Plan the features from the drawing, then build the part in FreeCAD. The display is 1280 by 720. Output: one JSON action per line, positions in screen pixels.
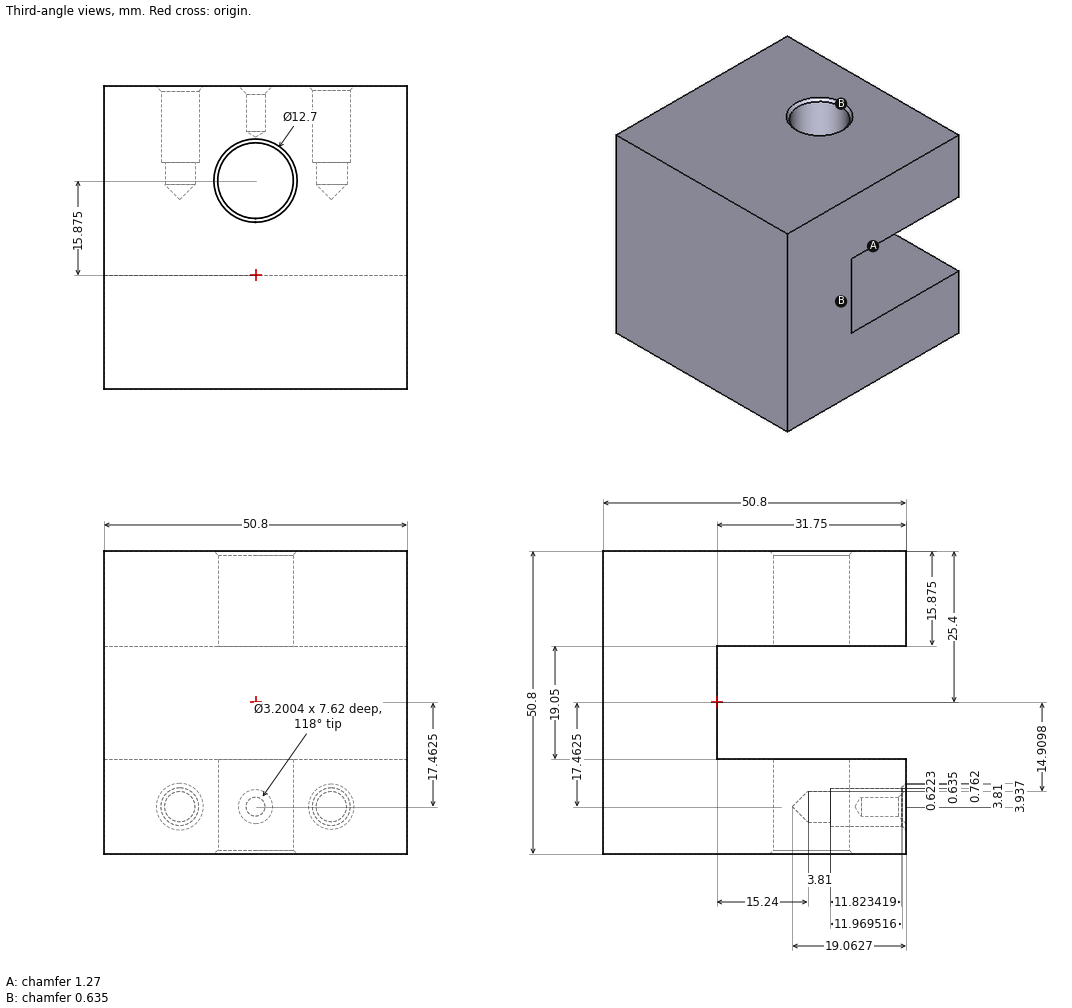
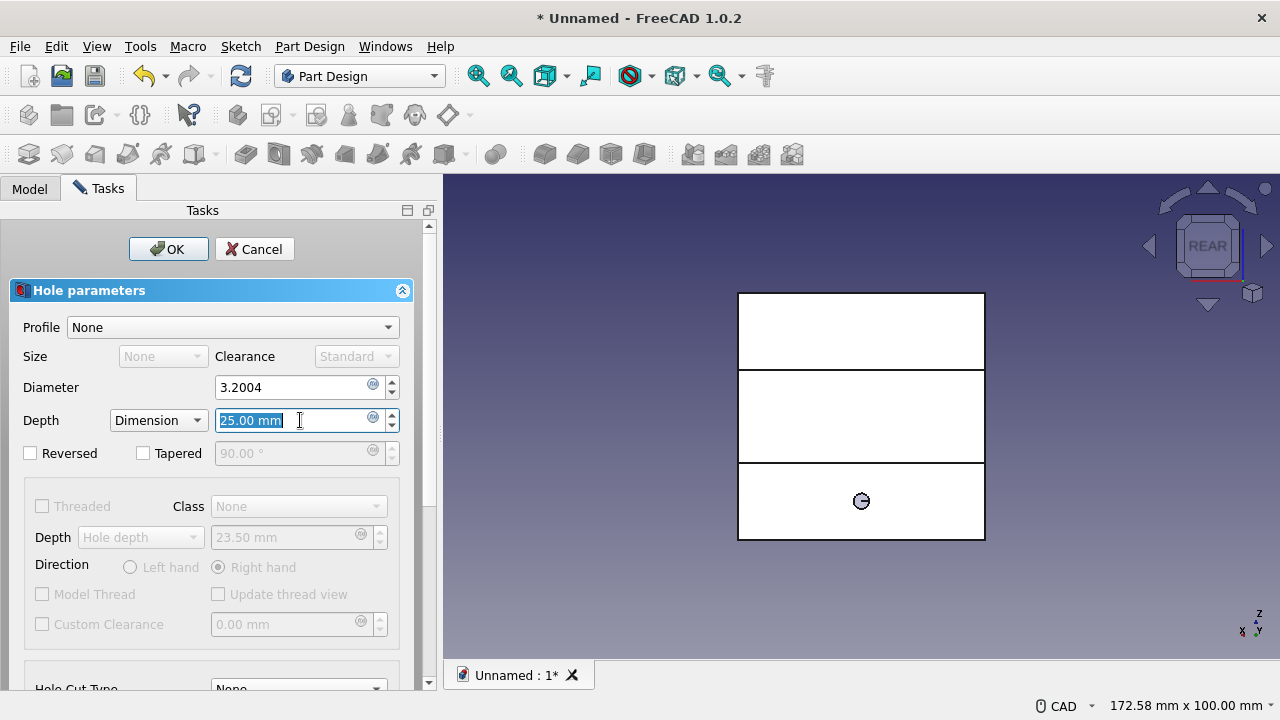
{"action": "type", "text": "7.62"}
{"action": "key", "text": "Tab"}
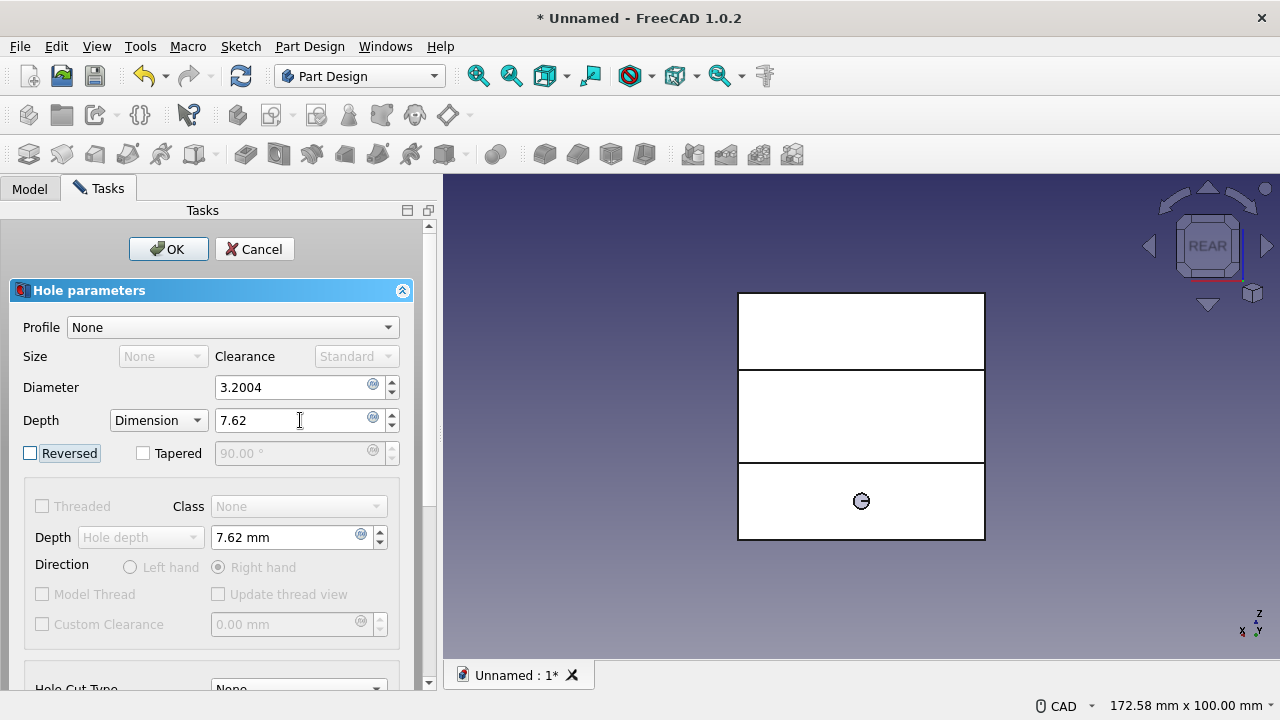
{"action": "left_click", "coordinate": [169, 249]}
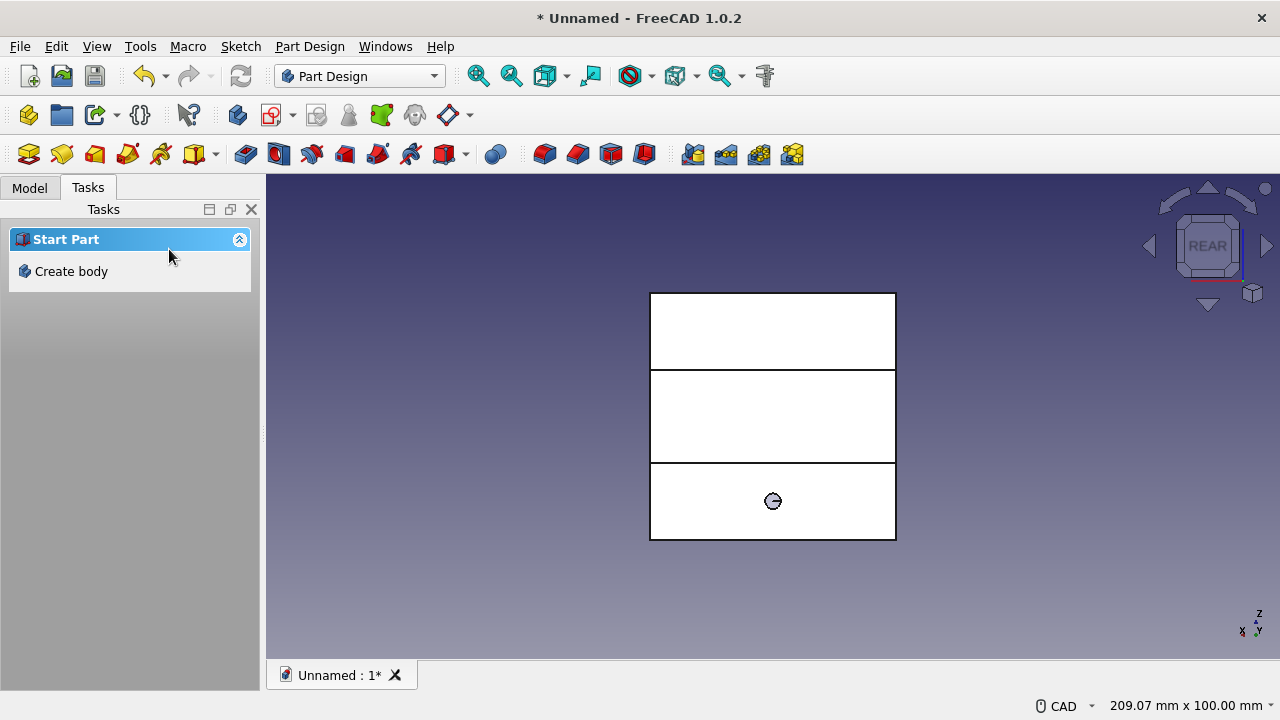
{"action": "left_click", "coordinate": [765, 500]}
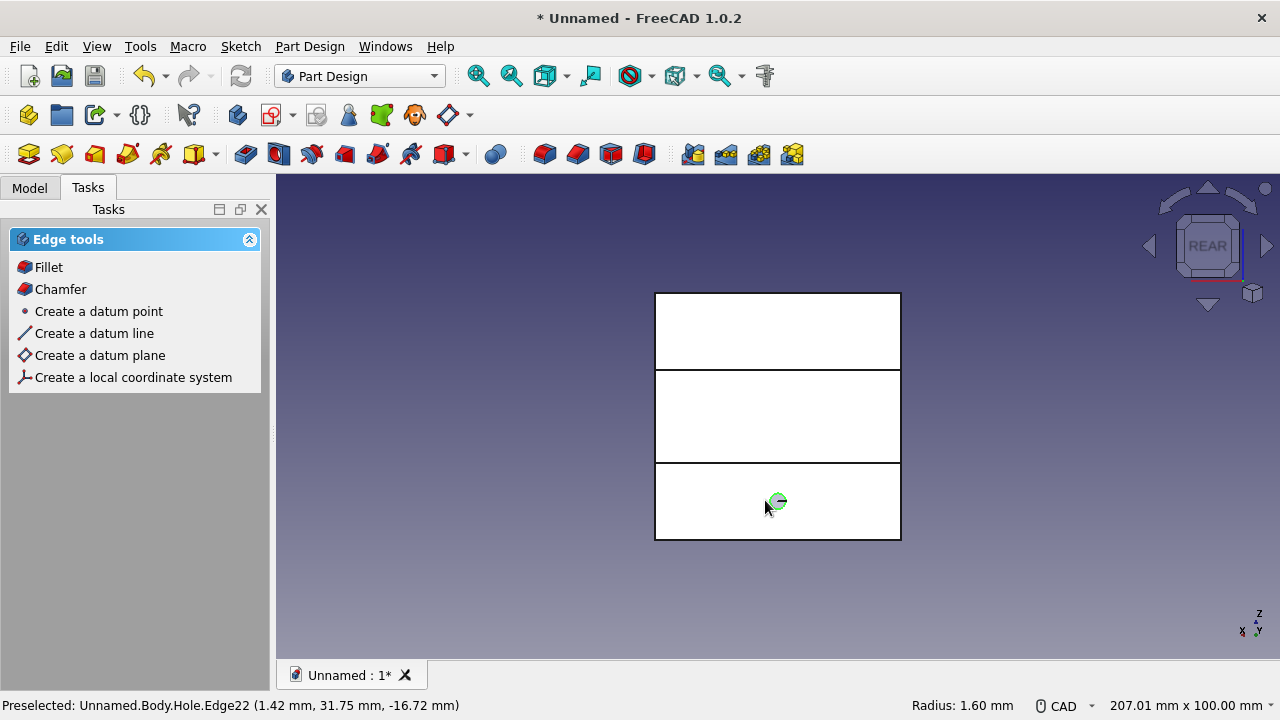
{"action": "left_click", "coordinate": [578, 154]}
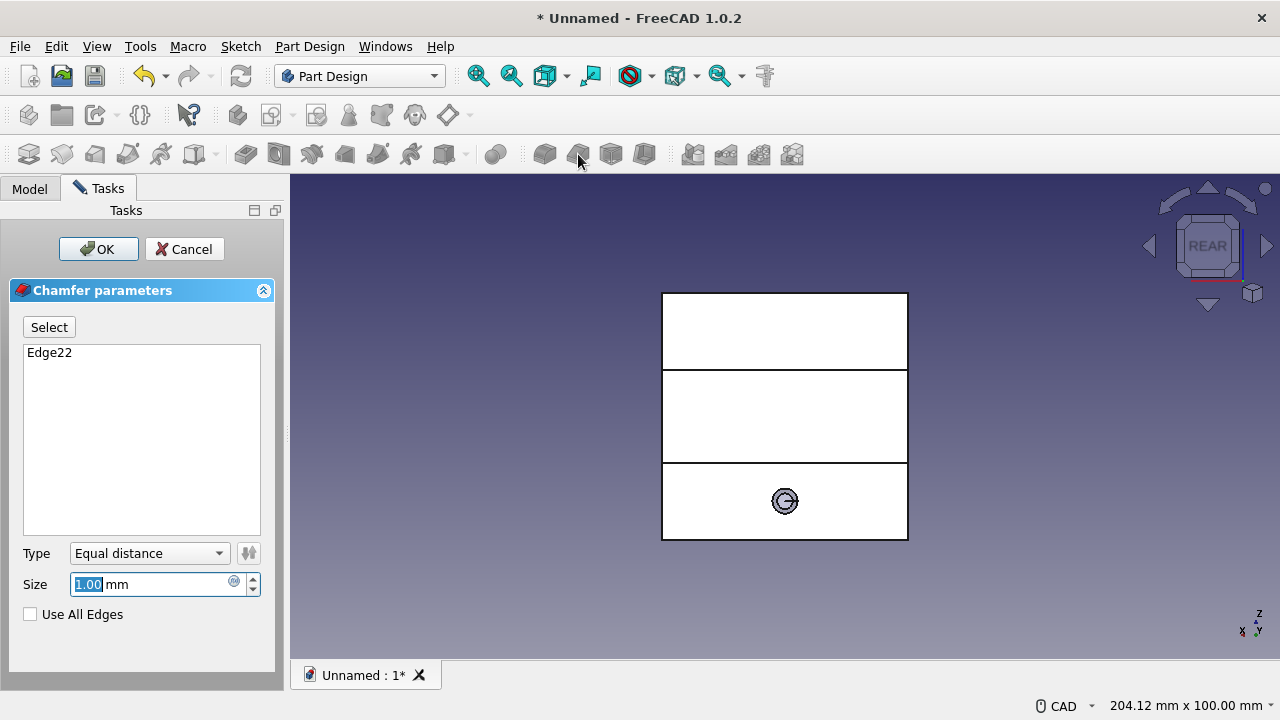
{"action": "type", "text": "1.27"}
{"action": "key", "text": "Tab"}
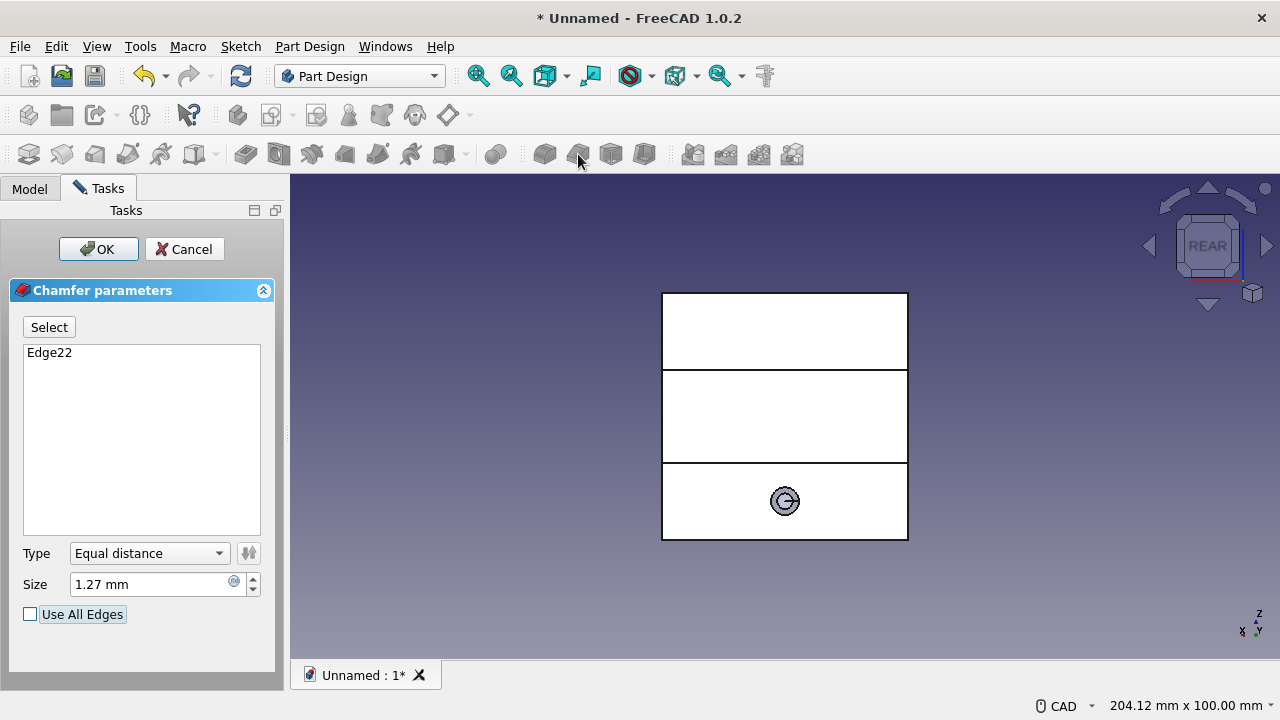
{"action": "left_click", "coordinate": [99, 249]}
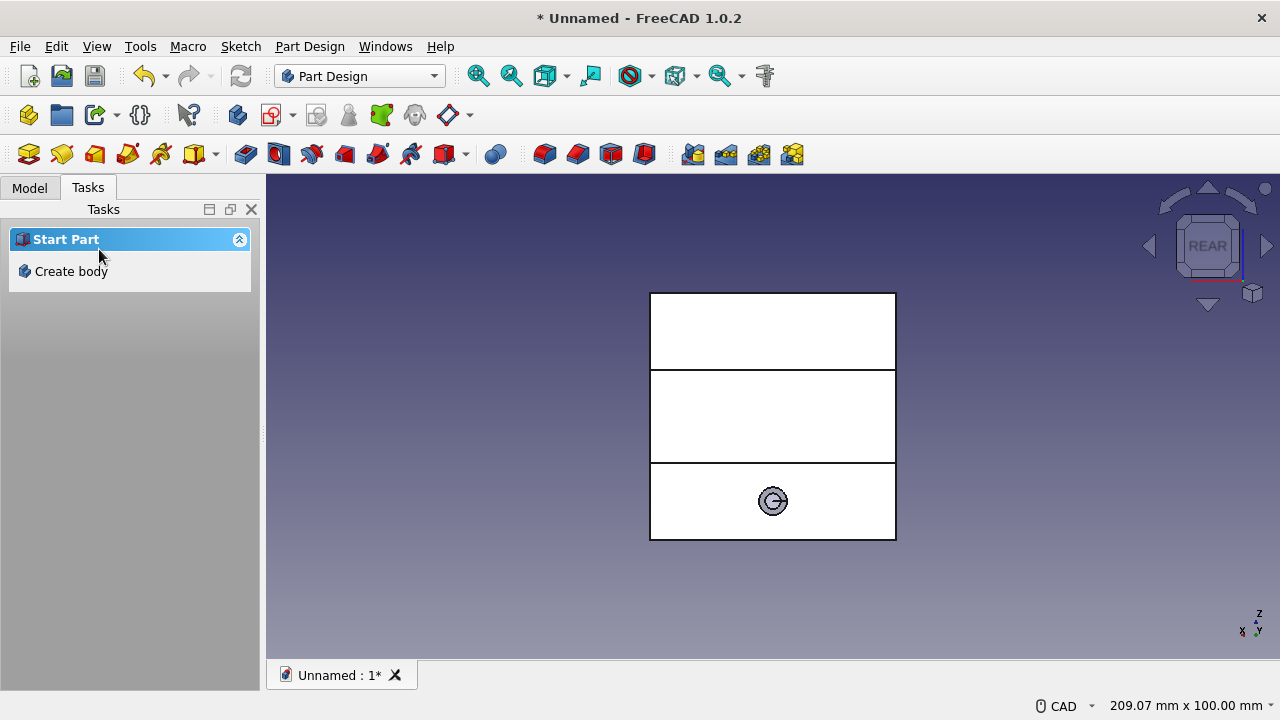
{"action": "left_click", "coordinate": [30, 188]}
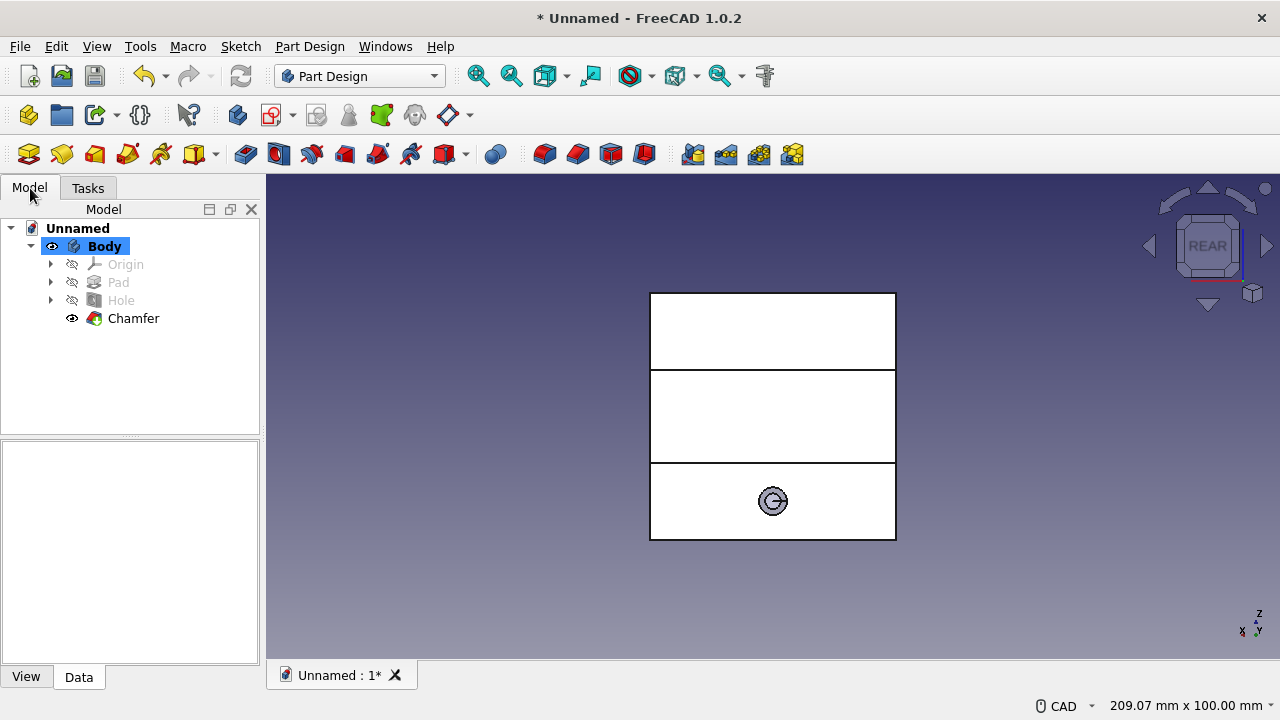
{"action": "left_click", "coordinate": [51, 264]}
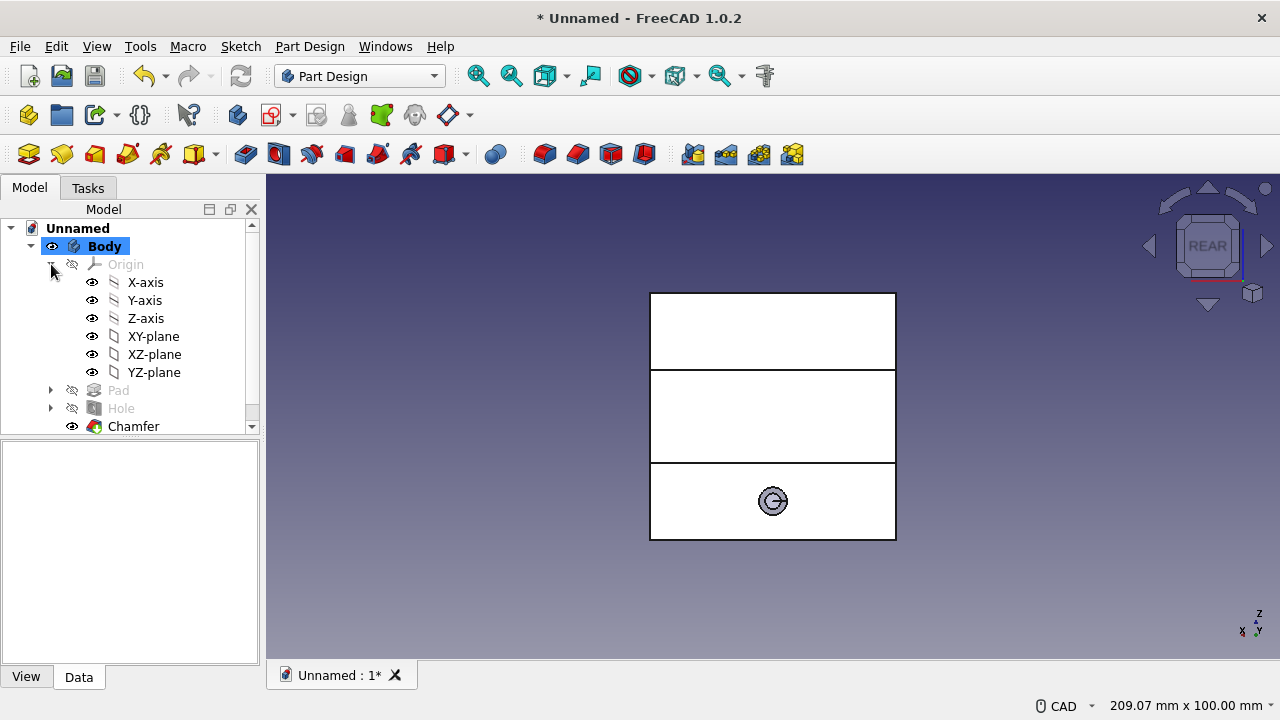
{"action": "left_click", "coordinate": [137, 372]}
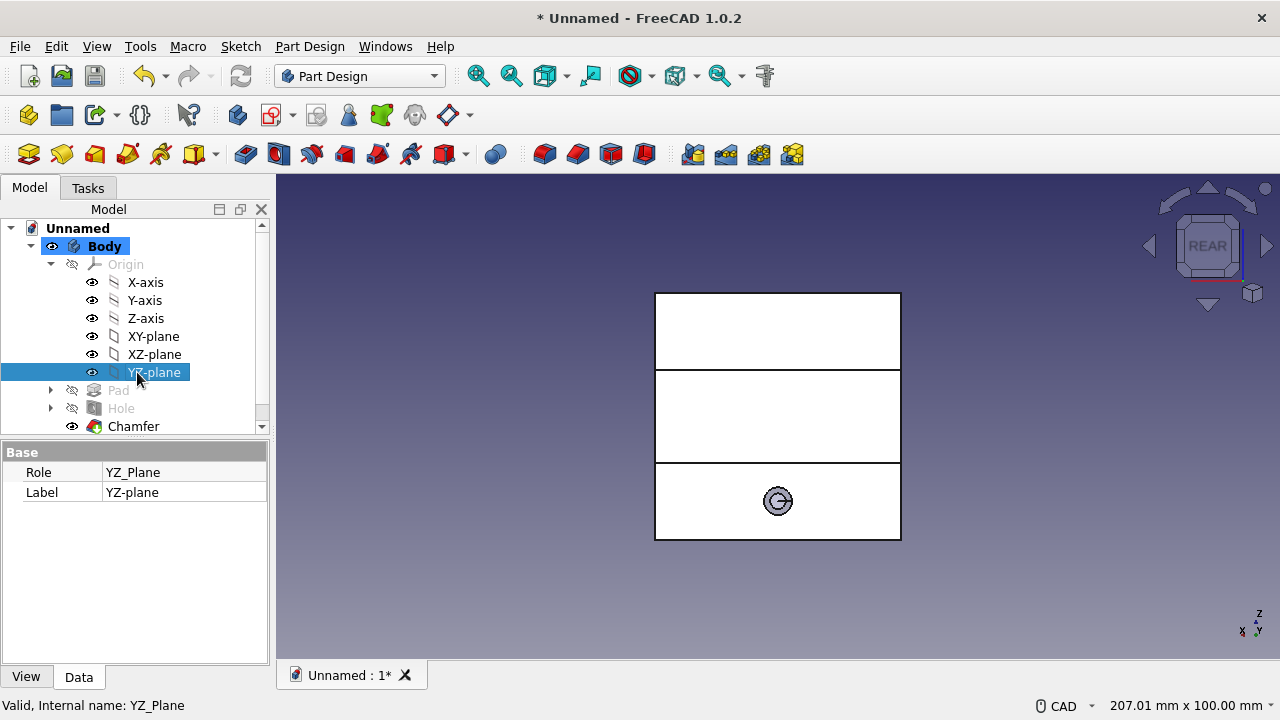
{"action": "left_click", "coordinate": [448, 116]}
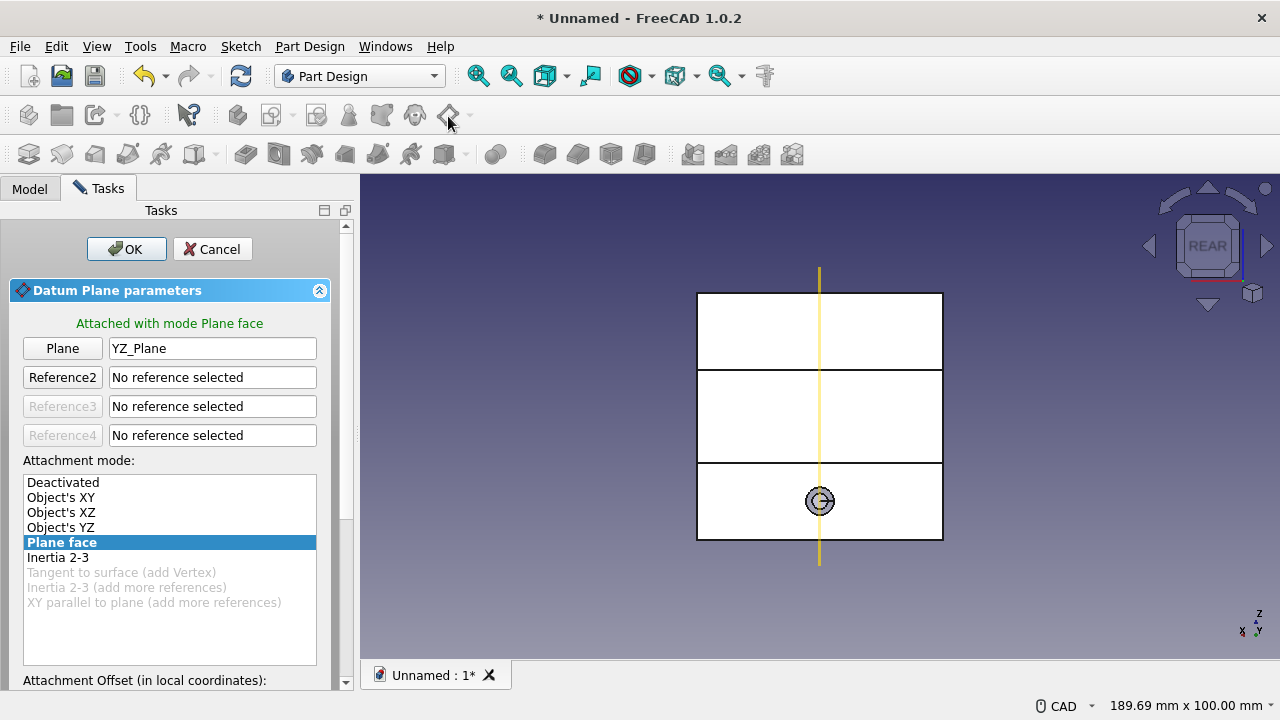
{"action": "scroll", "coordinate": [346, 455], "scroll_direction": "down", "scroll_amount": 3}